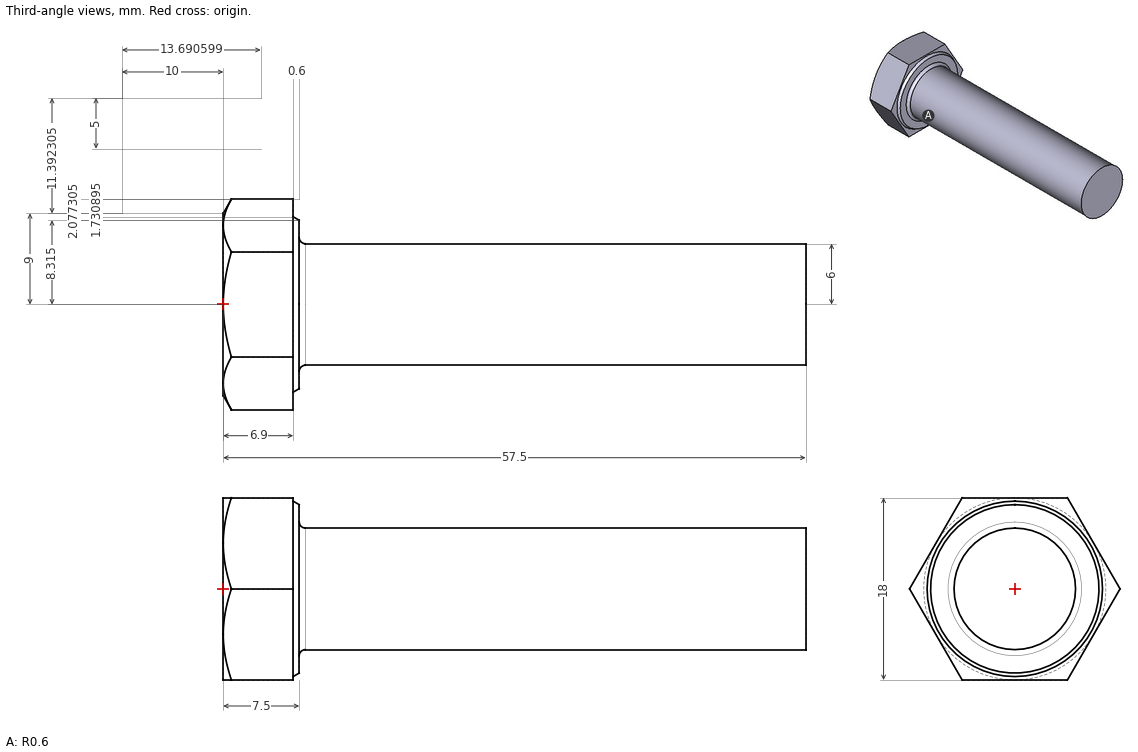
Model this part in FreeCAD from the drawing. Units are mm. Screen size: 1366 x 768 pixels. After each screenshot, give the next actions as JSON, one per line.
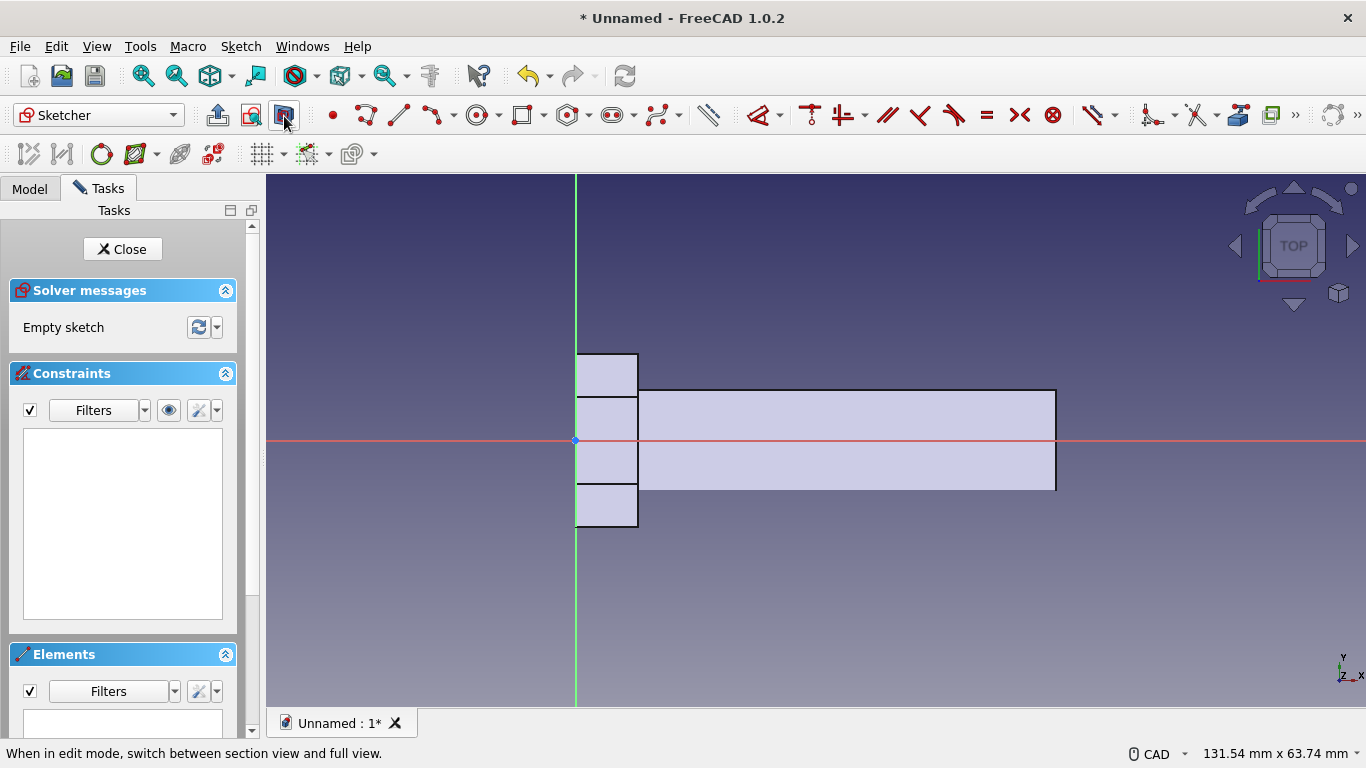
{"action": "scroll", "coordinate": [308, 252], "scroll_direction": "up", "scroll_amount": 3}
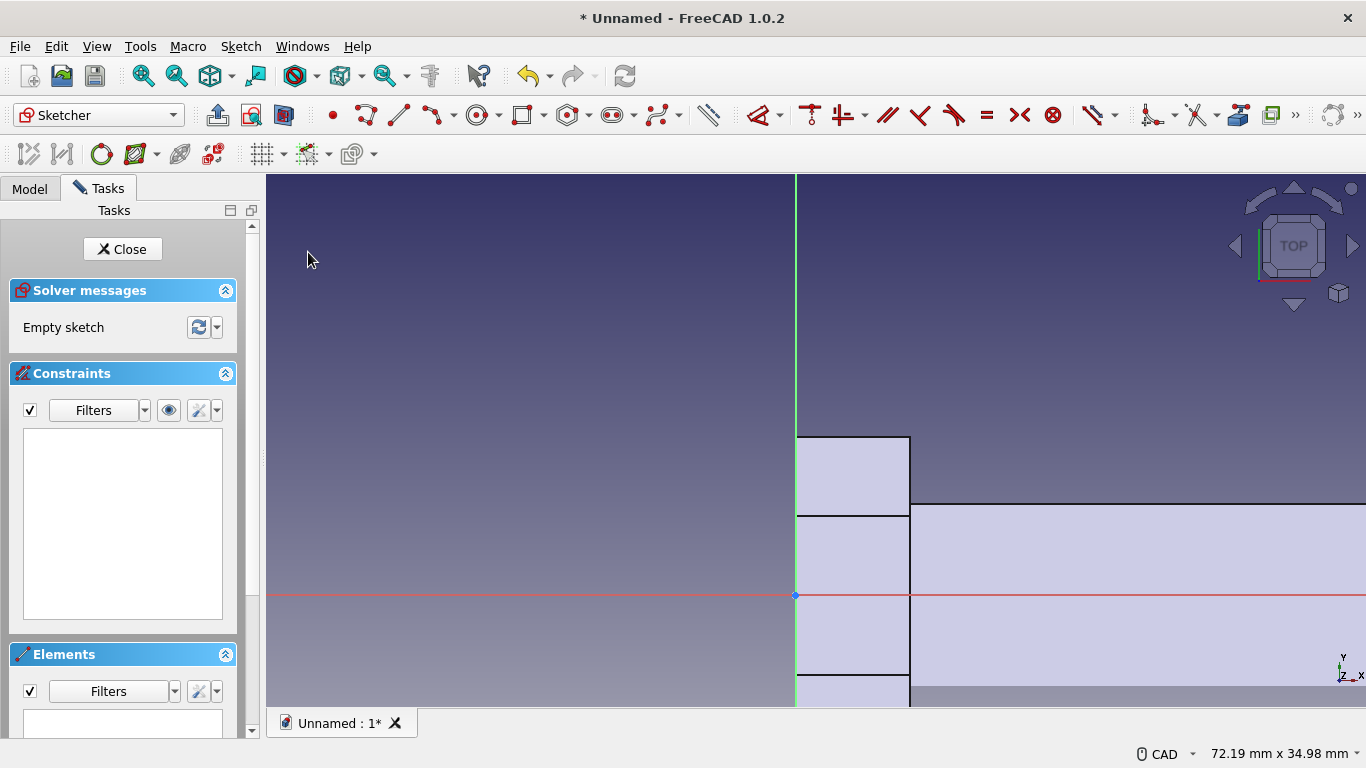
{"action": "left_click", "coordinate": [366, 116]}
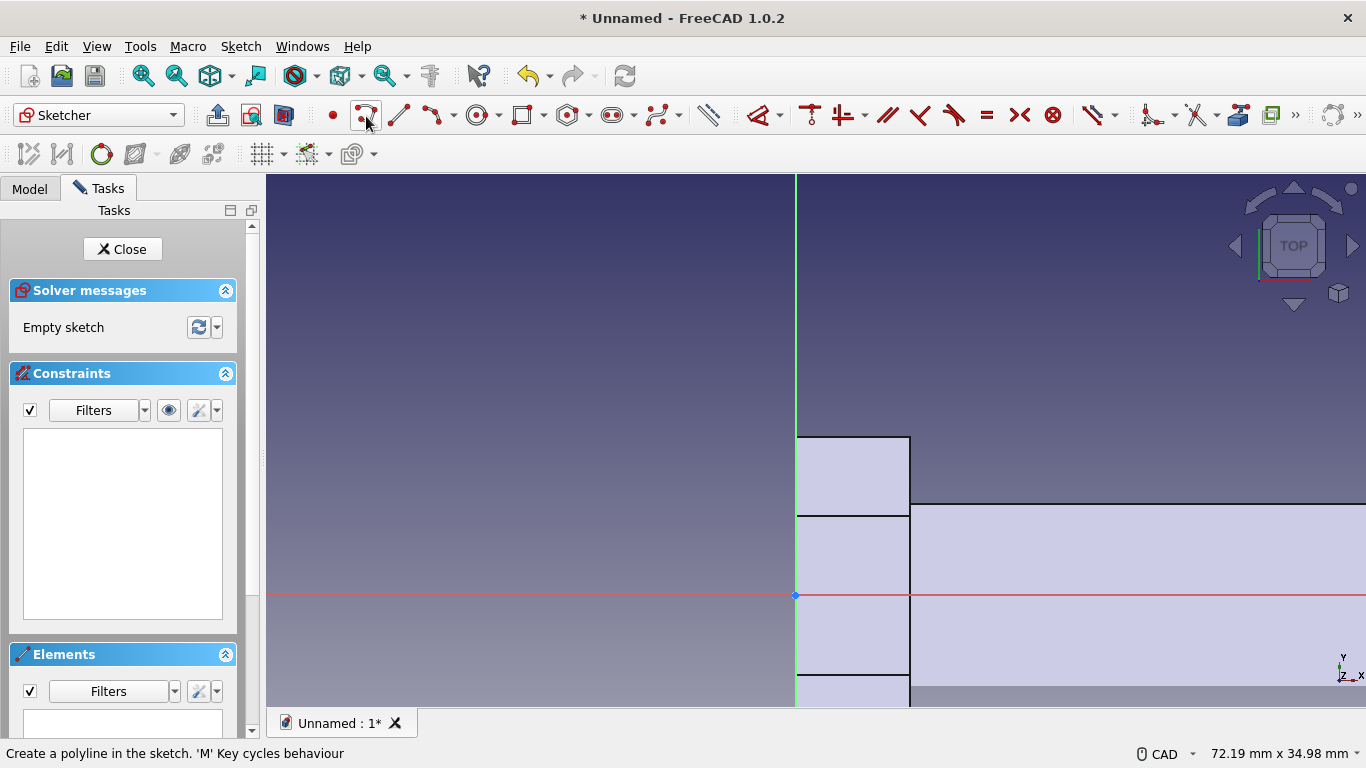
{"action": "left_click", "coordinate": [796, 458]}
{"action": "left_click", "coordinate": [852, 361]}
{"action": "left_click", "coordinate": [852, 285]}
{"action": "left_click", "coordinate": [643, 285]}
{"action": "left_click", "coordinate": [643, 458]}
{"action": "left_click", "coordinate": [796, 459]}
{"action": "key", "text": "Escape"}
{"action": "key", "text": "Escape"}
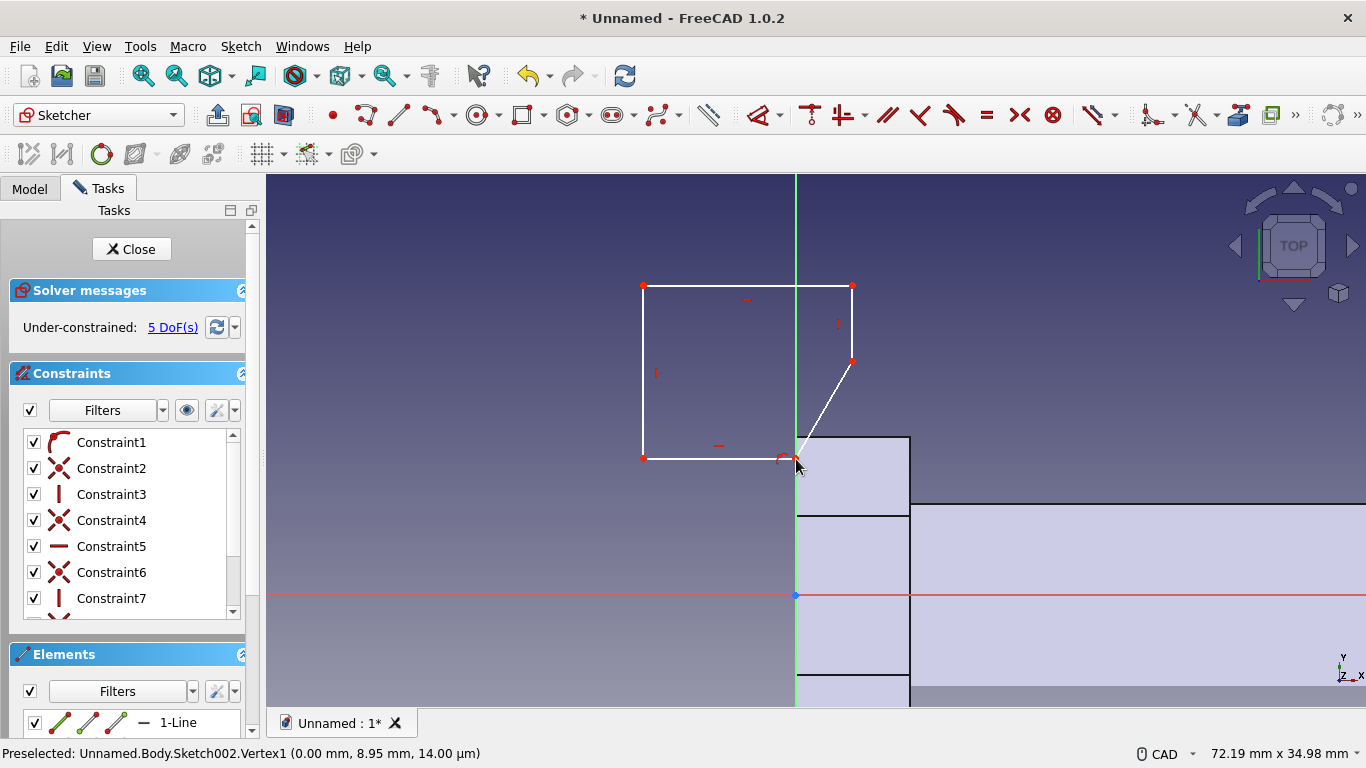
{"action": "left_click", "coordinate": [758, 116]}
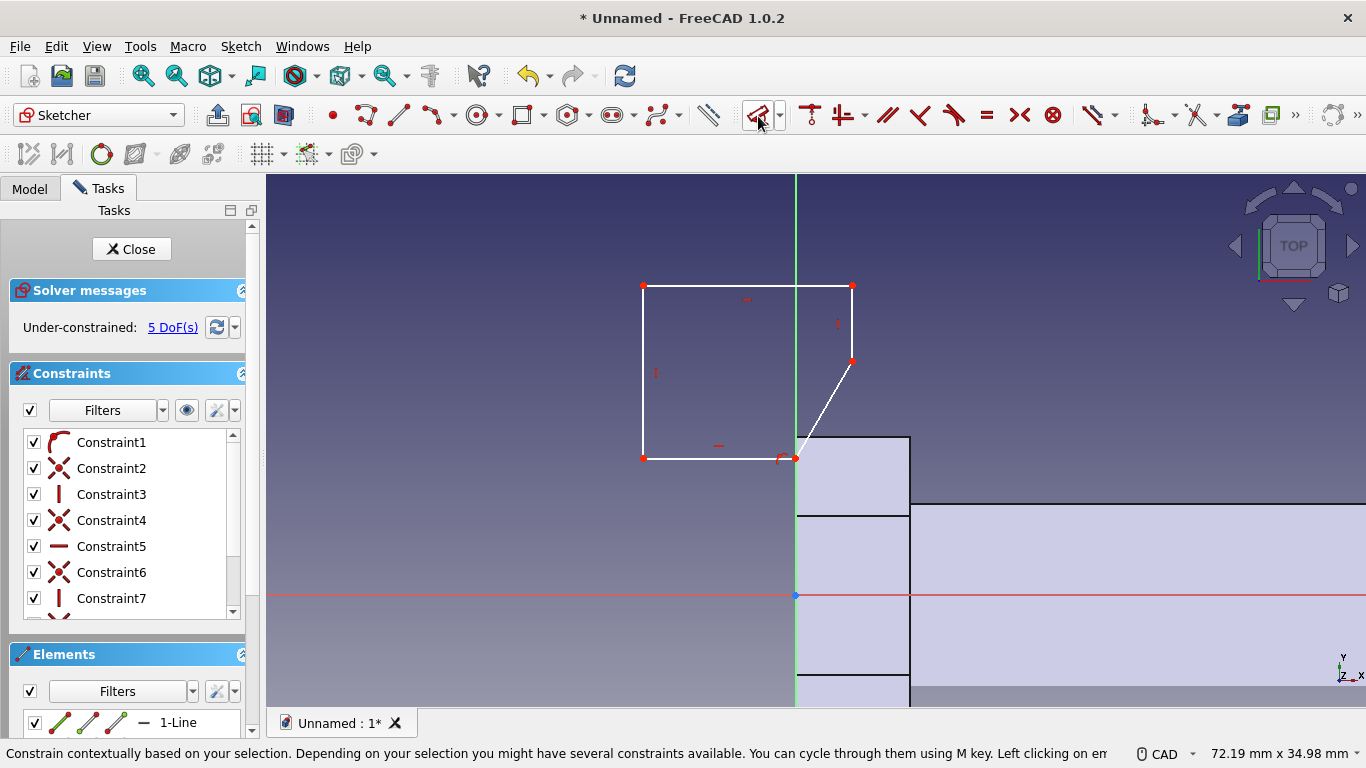
{"action": "left_click", "coordinate": [852, 339]}
{"action": "left_click", "coordinate": [886, 324]}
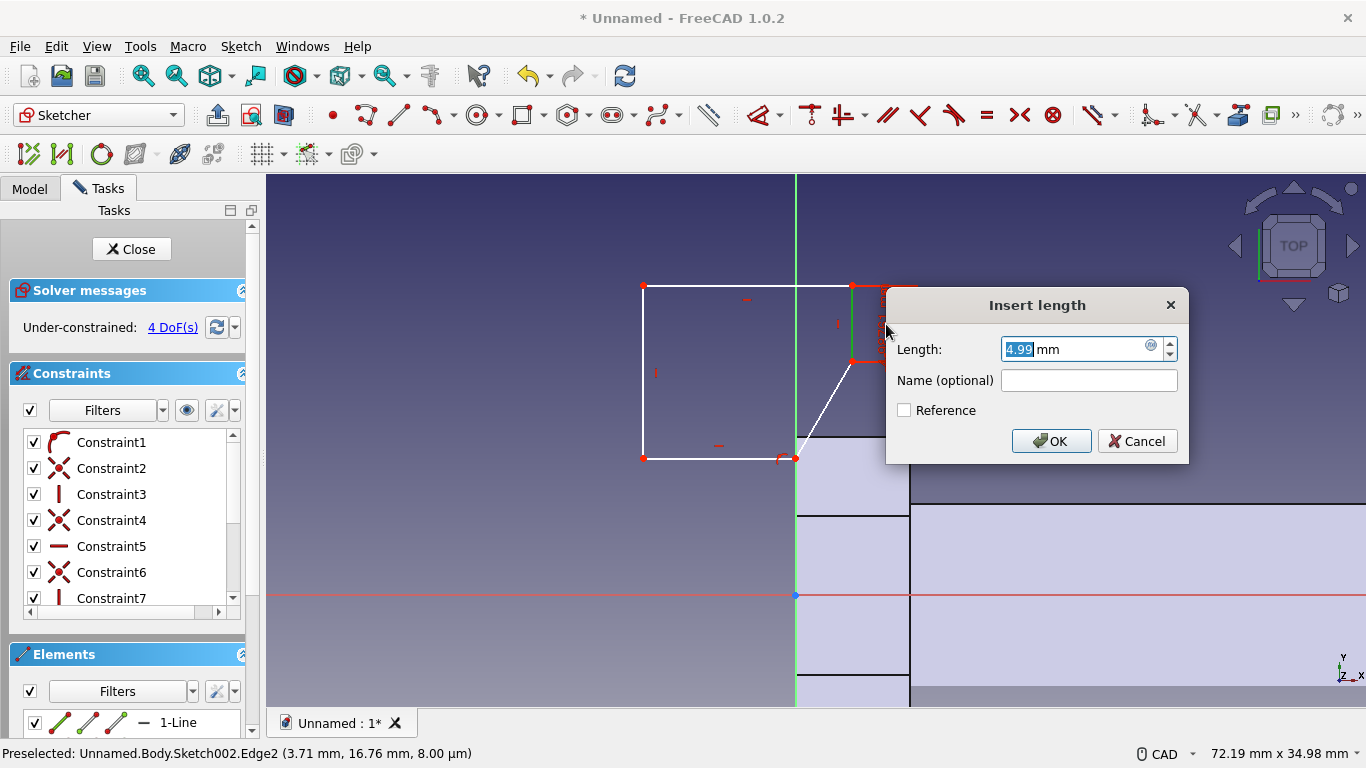
{"action": "type", "text": "5"}
{"action": "key", "text": "Return"}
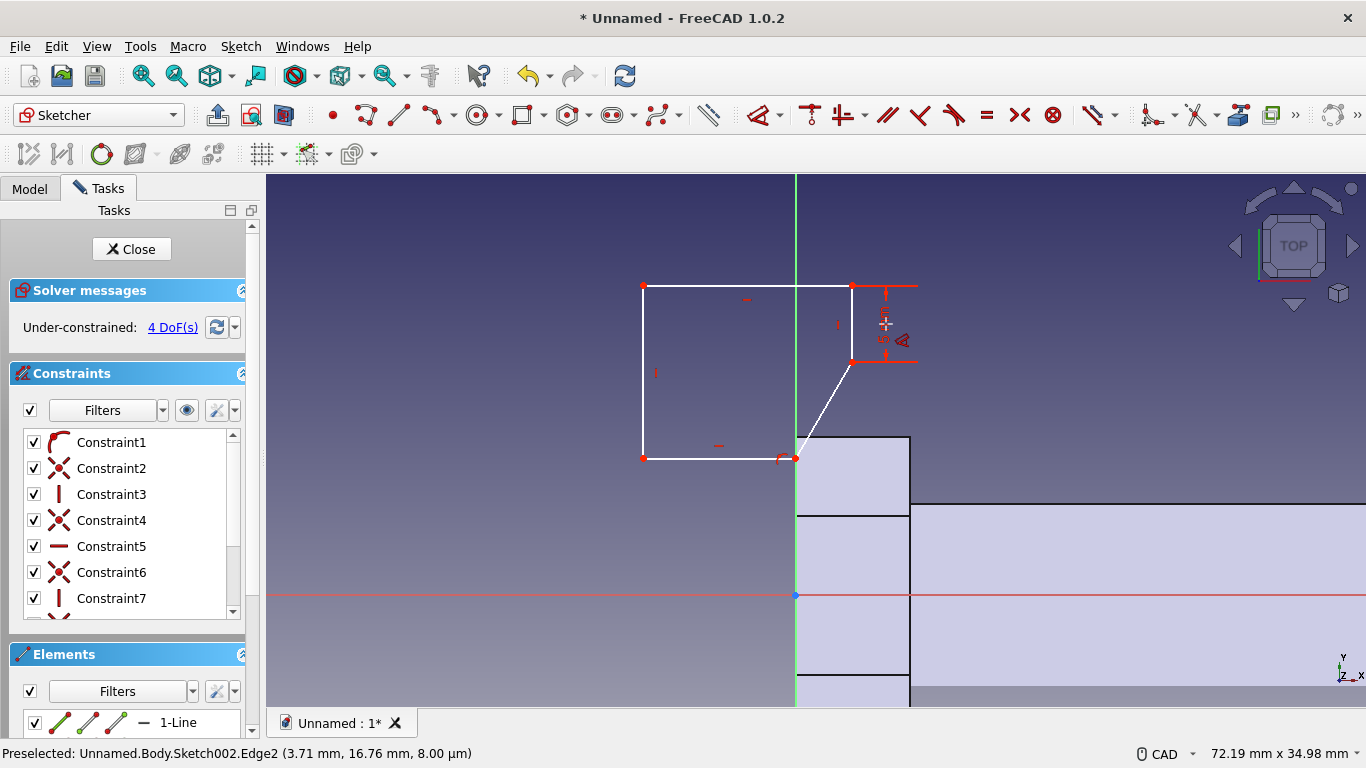
{"action": "left_click", "coordinate": [689, 459]}
{"action": "left_click", "coordinate": [719, 493]}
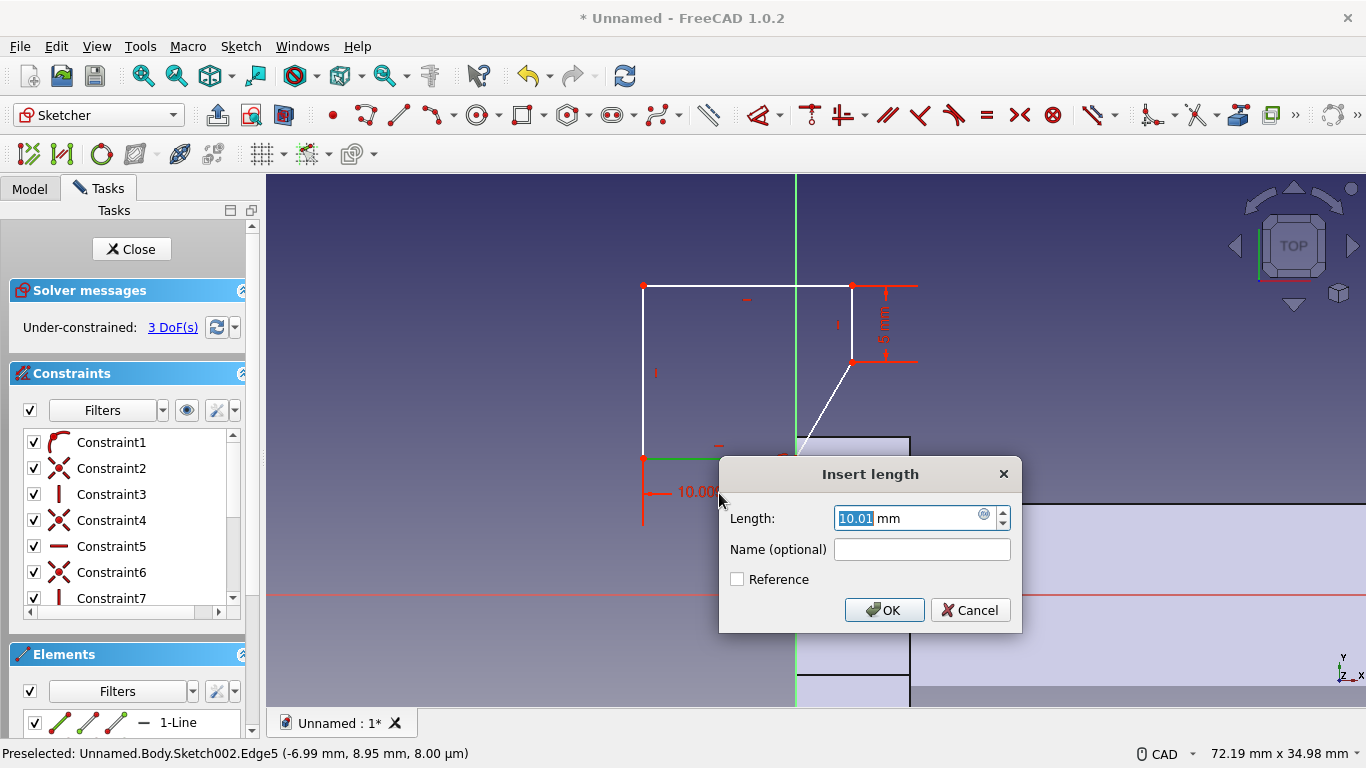
{"action": "type", "text": "10"}
{"action": "key", "text": "Return"}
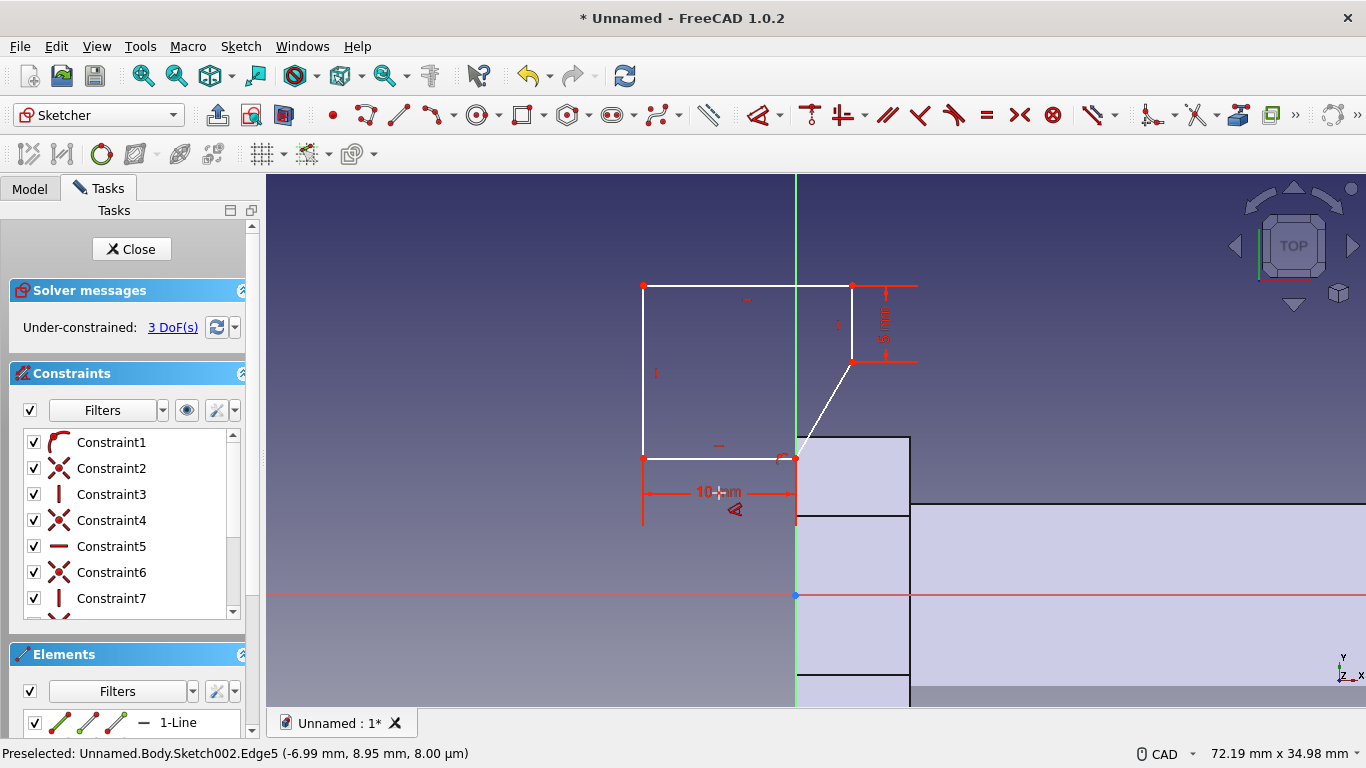
{"action": "left_click", "coordinate": [796, 459]}
{"action": "left_click", "coordinate": [830, 527]}